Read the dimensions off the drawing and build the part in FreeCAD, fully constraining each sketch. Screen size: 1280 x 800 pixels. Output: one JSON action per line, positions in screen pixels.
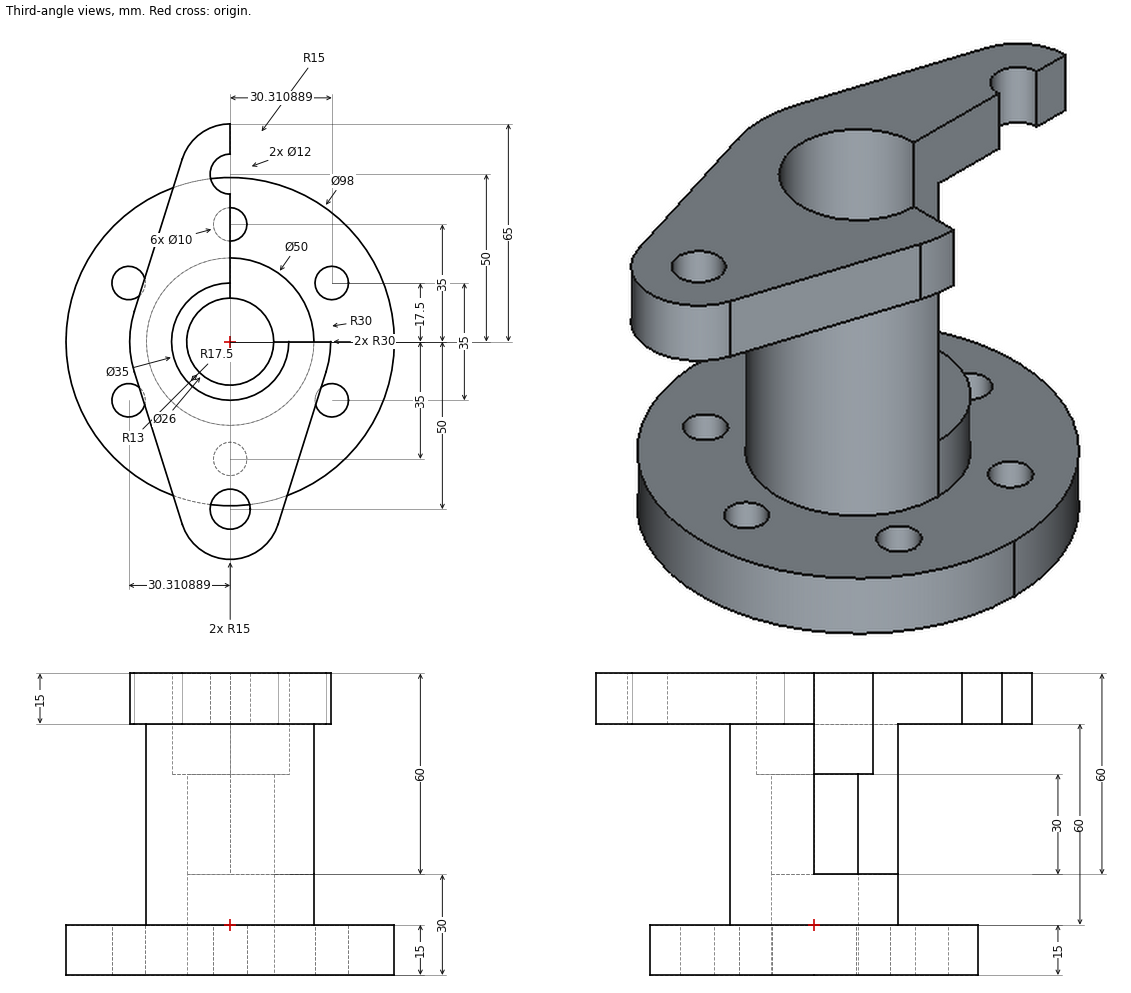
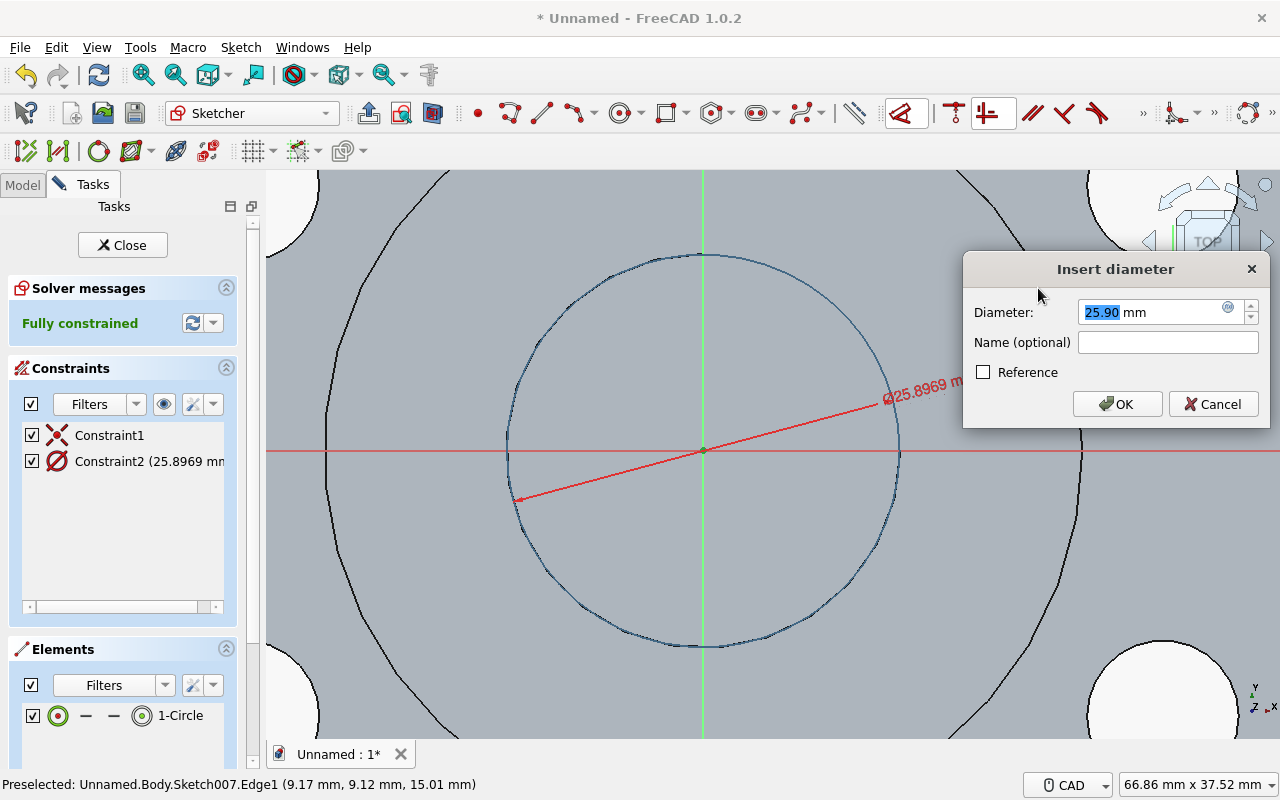
{"action": "type", "text": "26"}
{"action": "key", "text": "Return"}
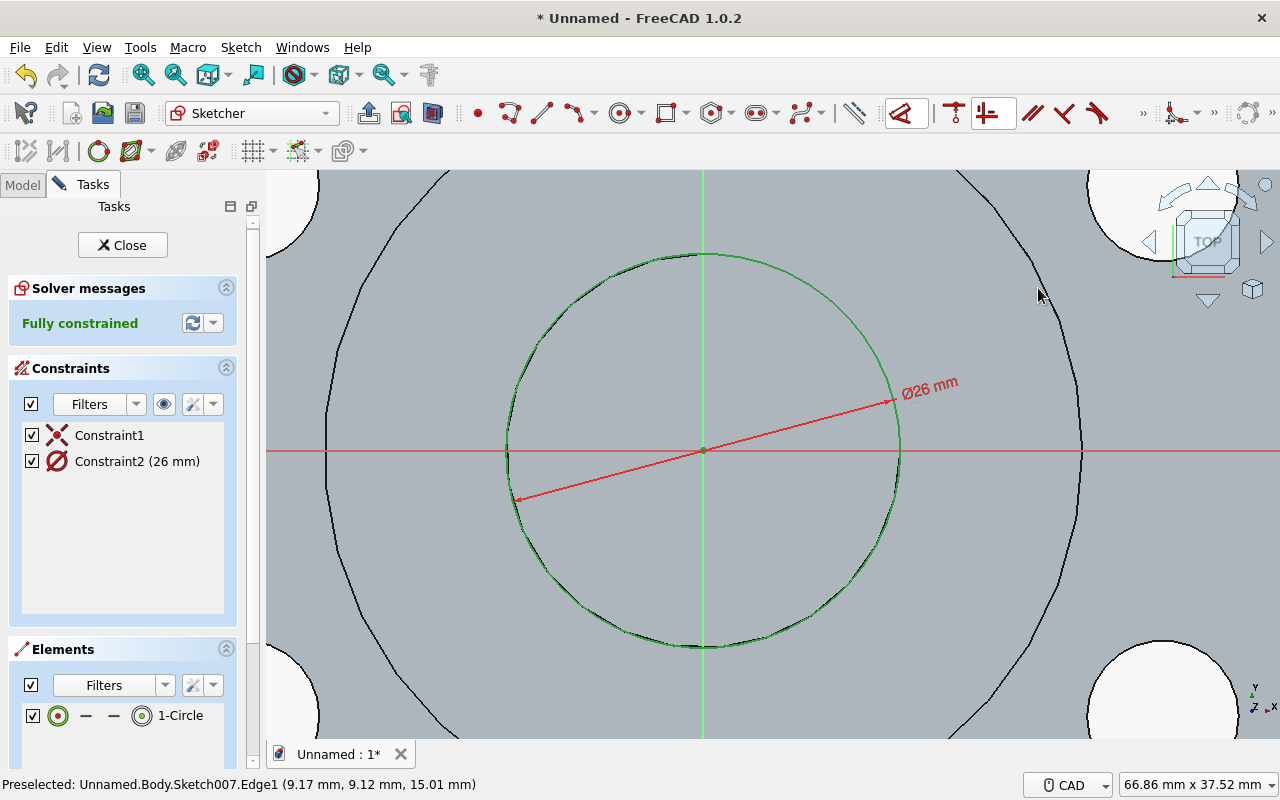
{"action": "left_click", "coordinate": [123, 245]}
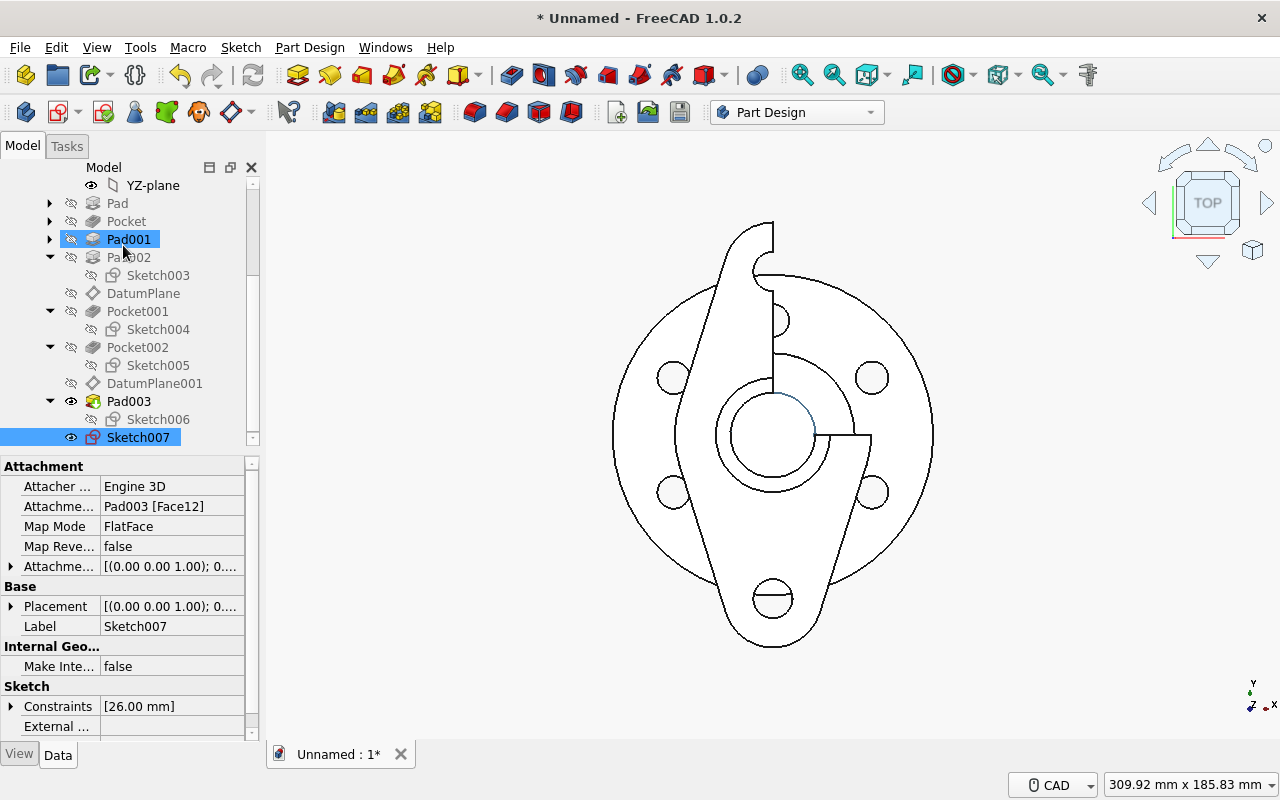
{"action": "left_click", "coordinate": [512, 76]}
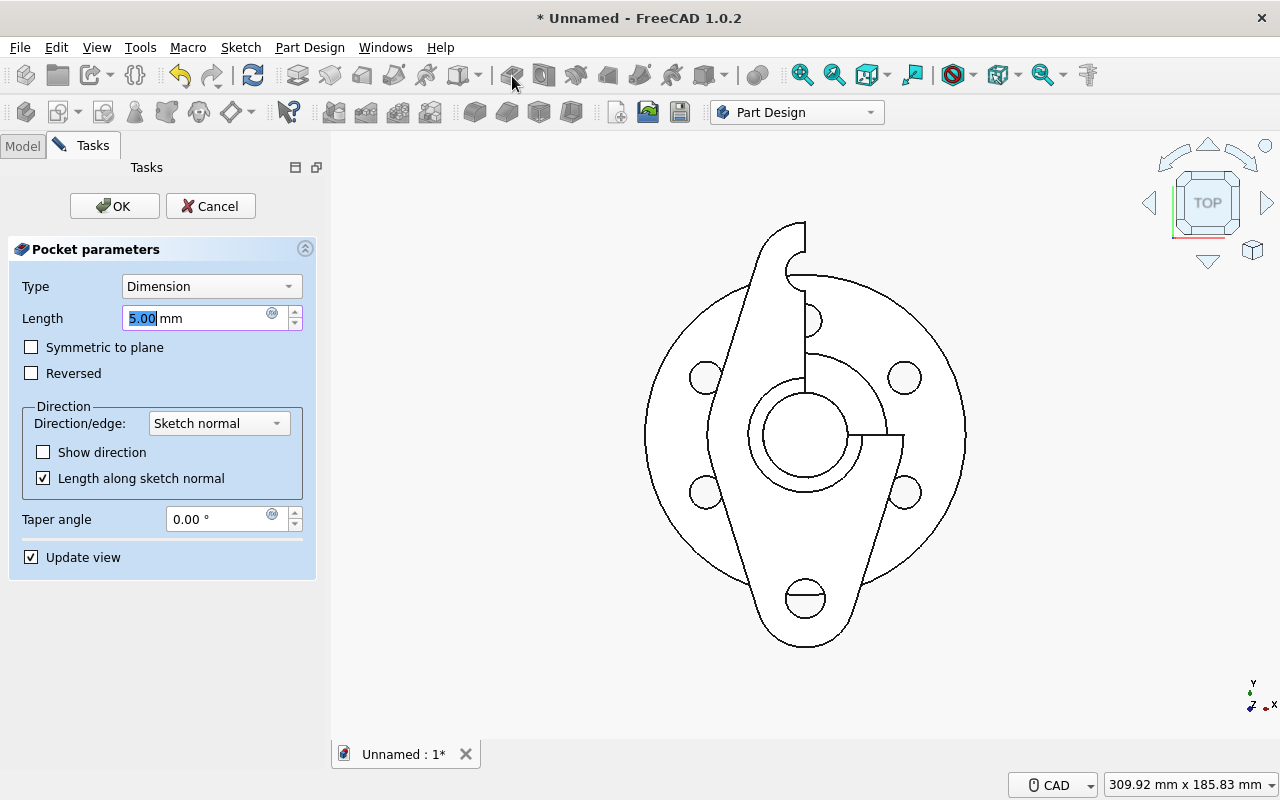
{"action": "type", "text": "30"}
{"action": "key", "text": "Tab"}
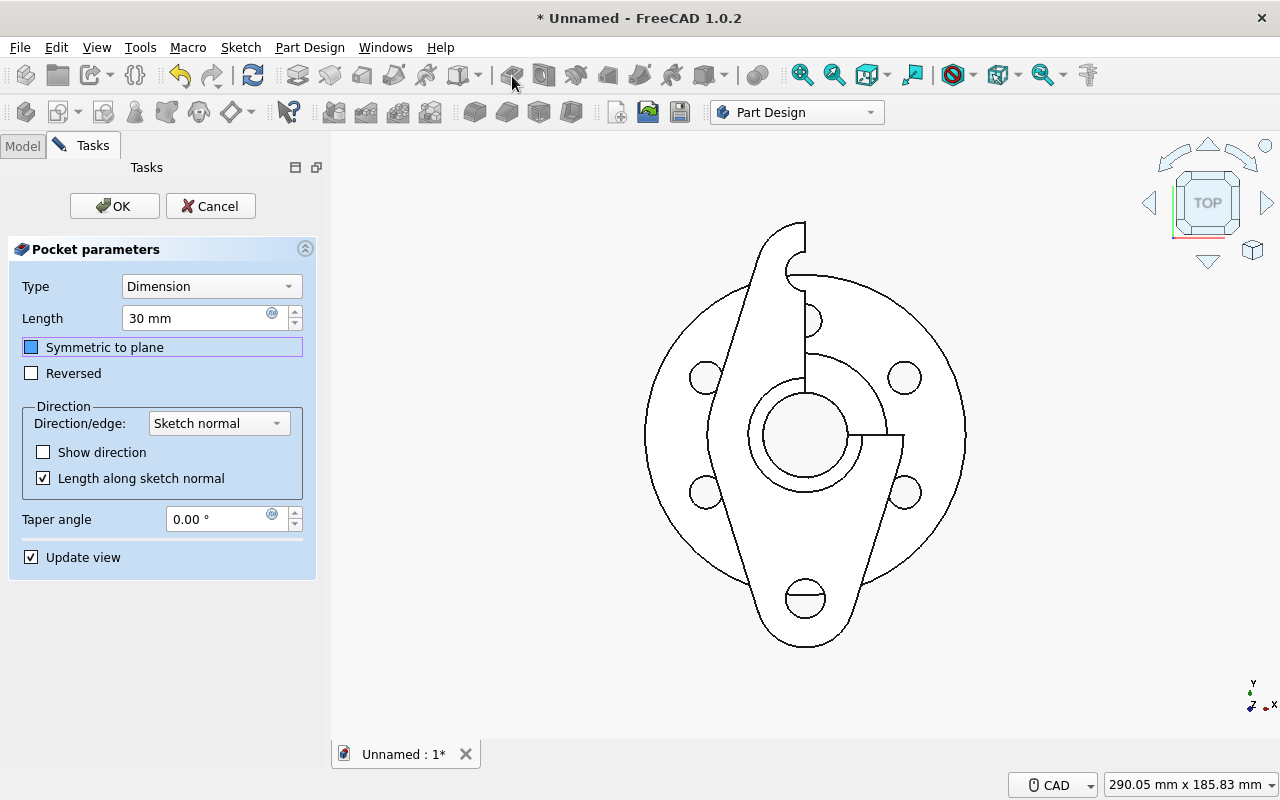
{"action": "left_click", "coordinate": [115, 206]}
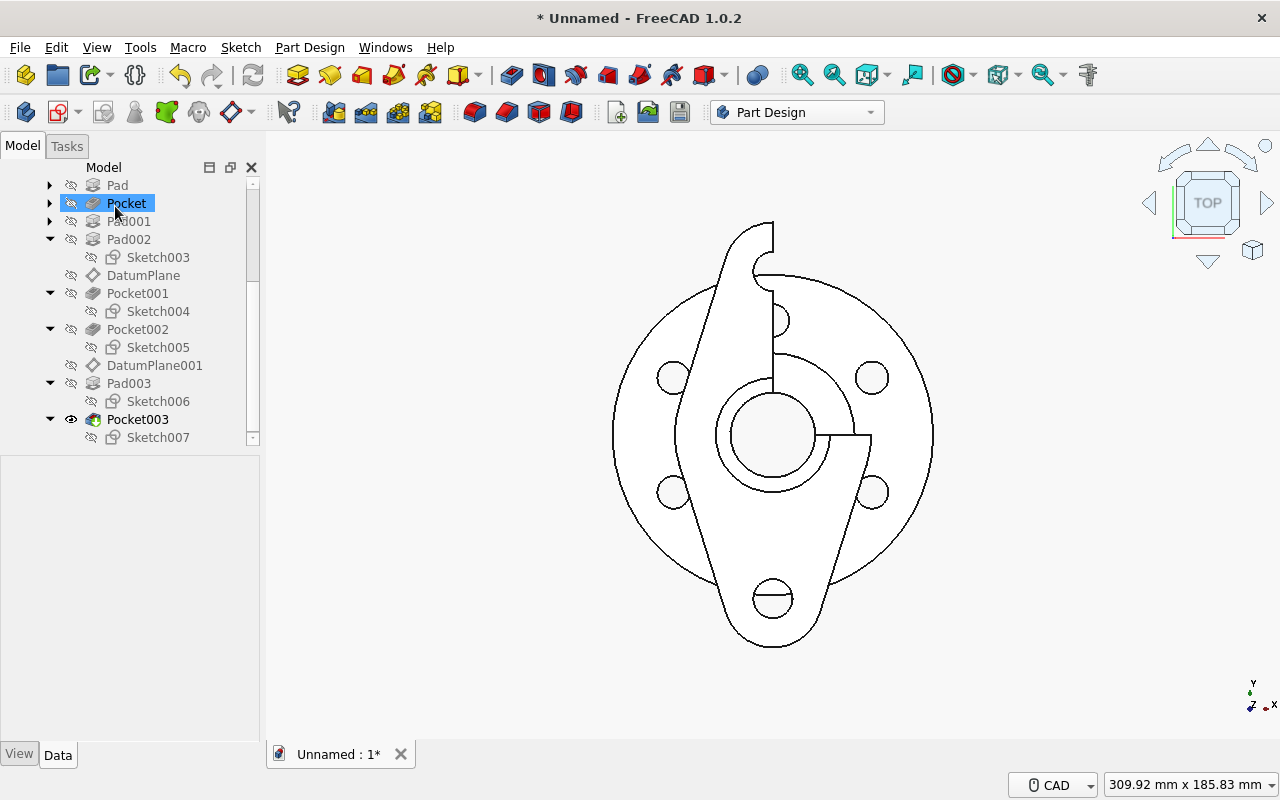
{"action": "key", "text": "0"}